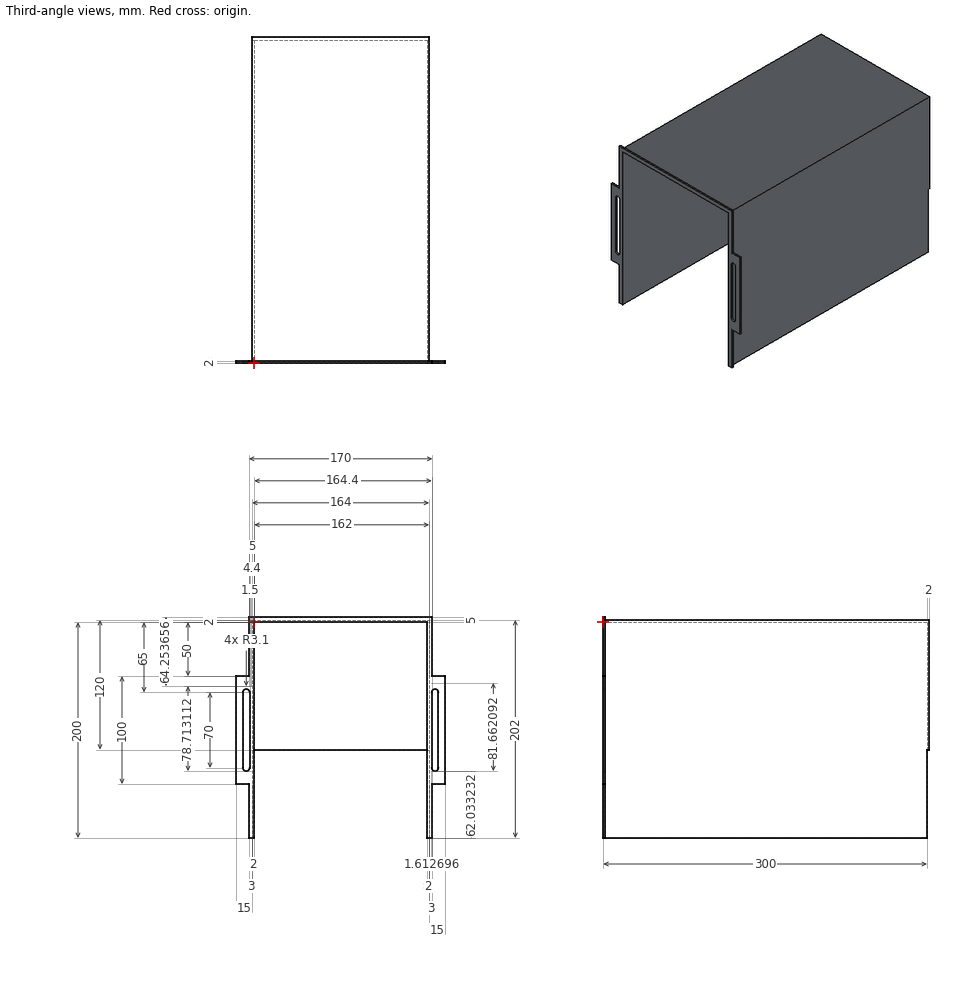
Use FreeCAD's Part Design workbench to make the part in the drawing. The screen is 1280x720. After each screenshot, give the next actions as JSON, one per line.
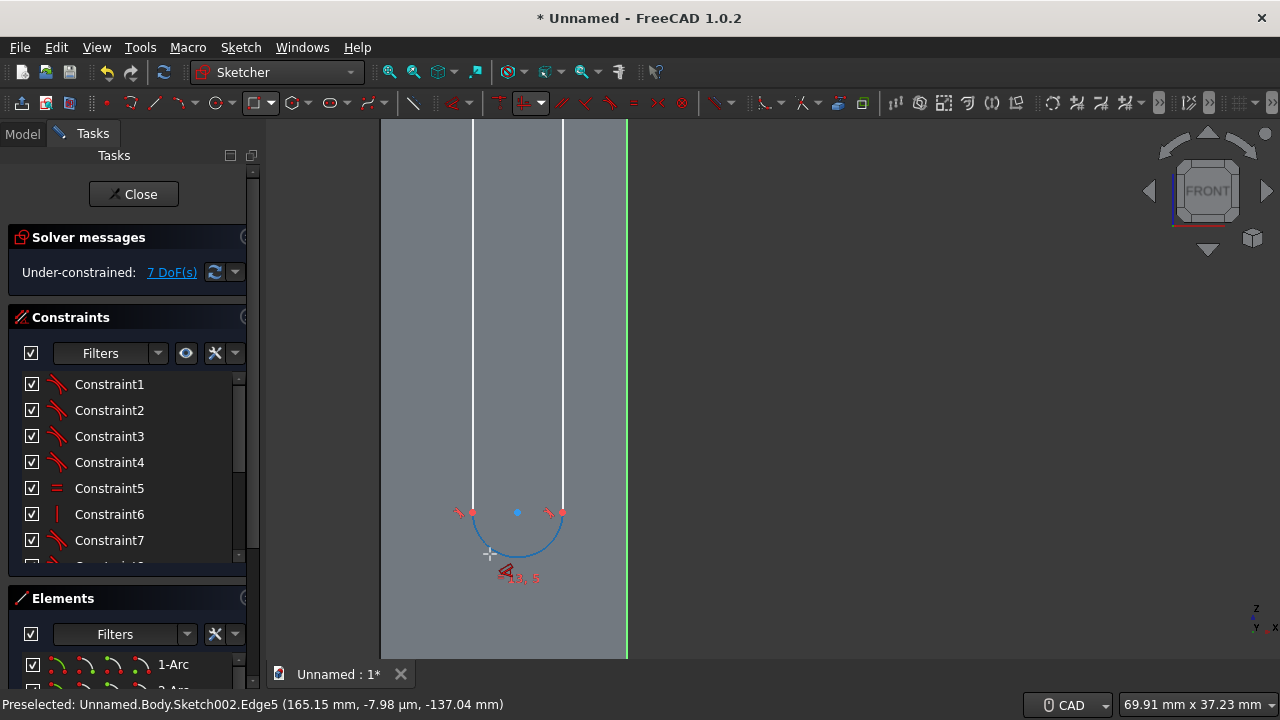
{"action": "left_click", "coordinate": [491, 549]}
{"action": "left_click", "coordinate": [472, 575]}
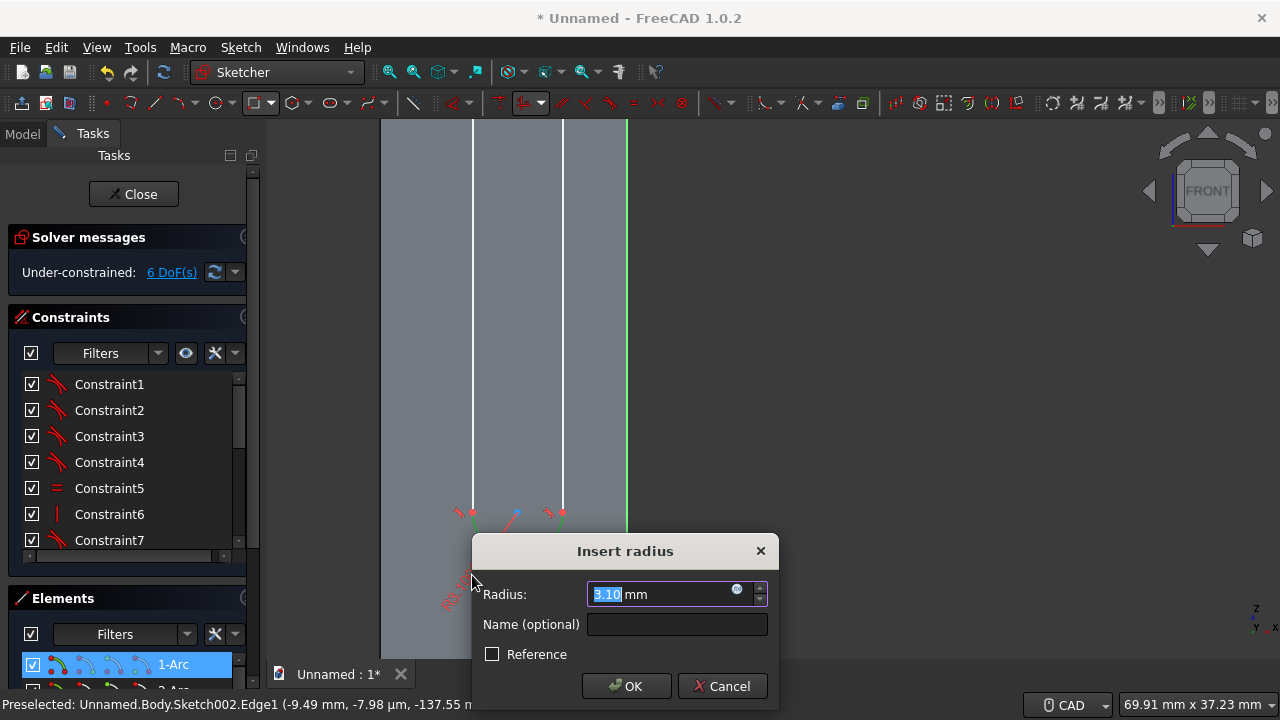
{"action": "type", "text": "3.1"}
{"action": "key", "text": "Return"}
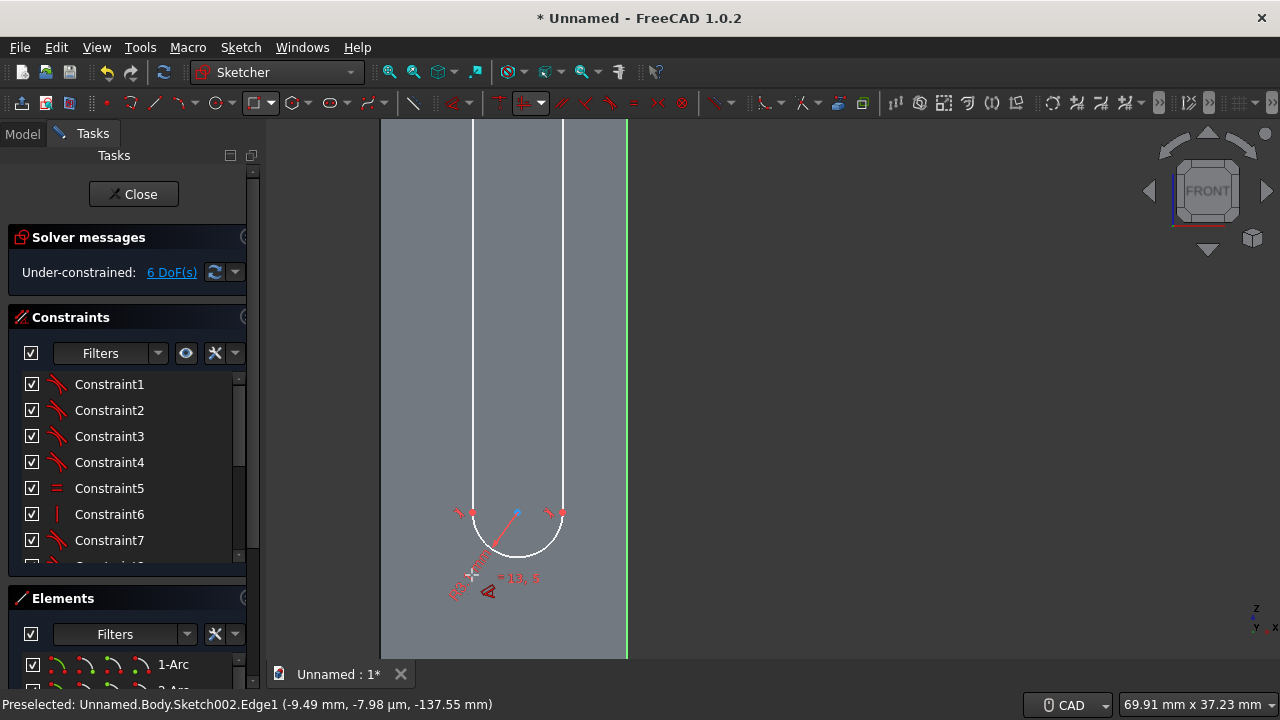
{"action": "scroll", "coordinate": [490, 554], "scroll_direction": "down", "scroll_amount": 9}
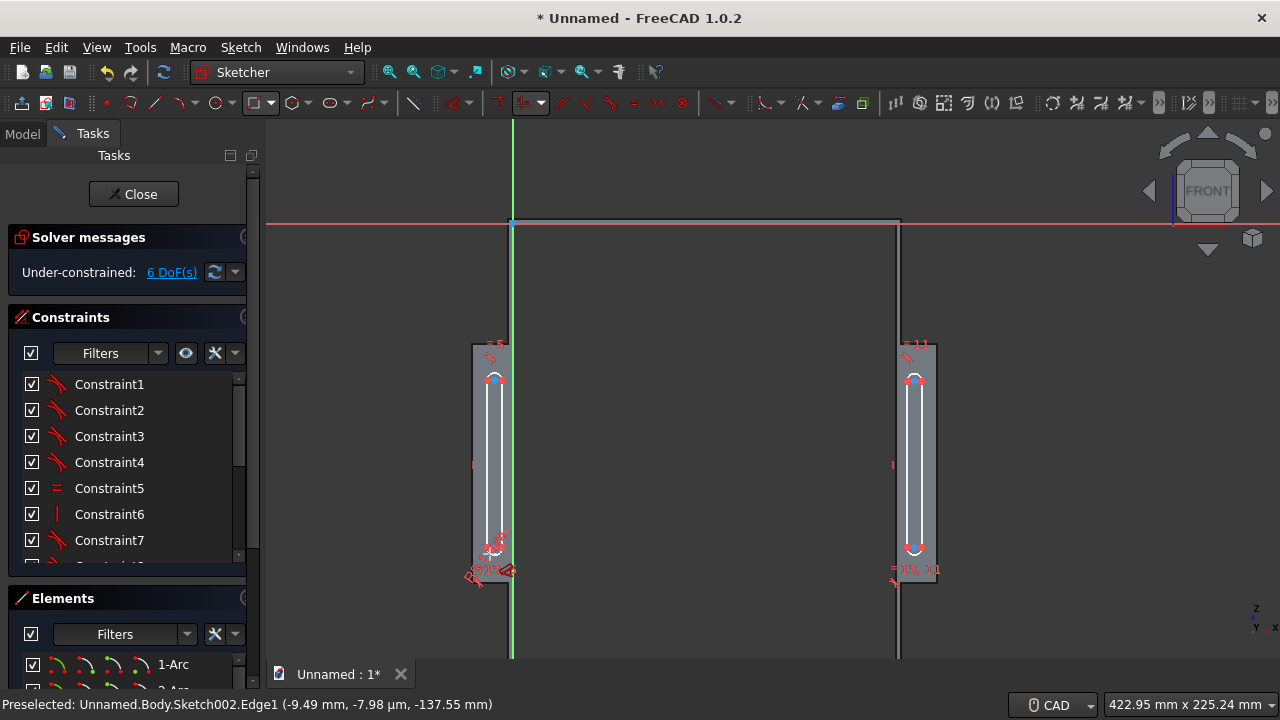
{"action": "left_click", "coordinate": [487, 498]}
{"action": "left_click", "coordinate": [453, 464]}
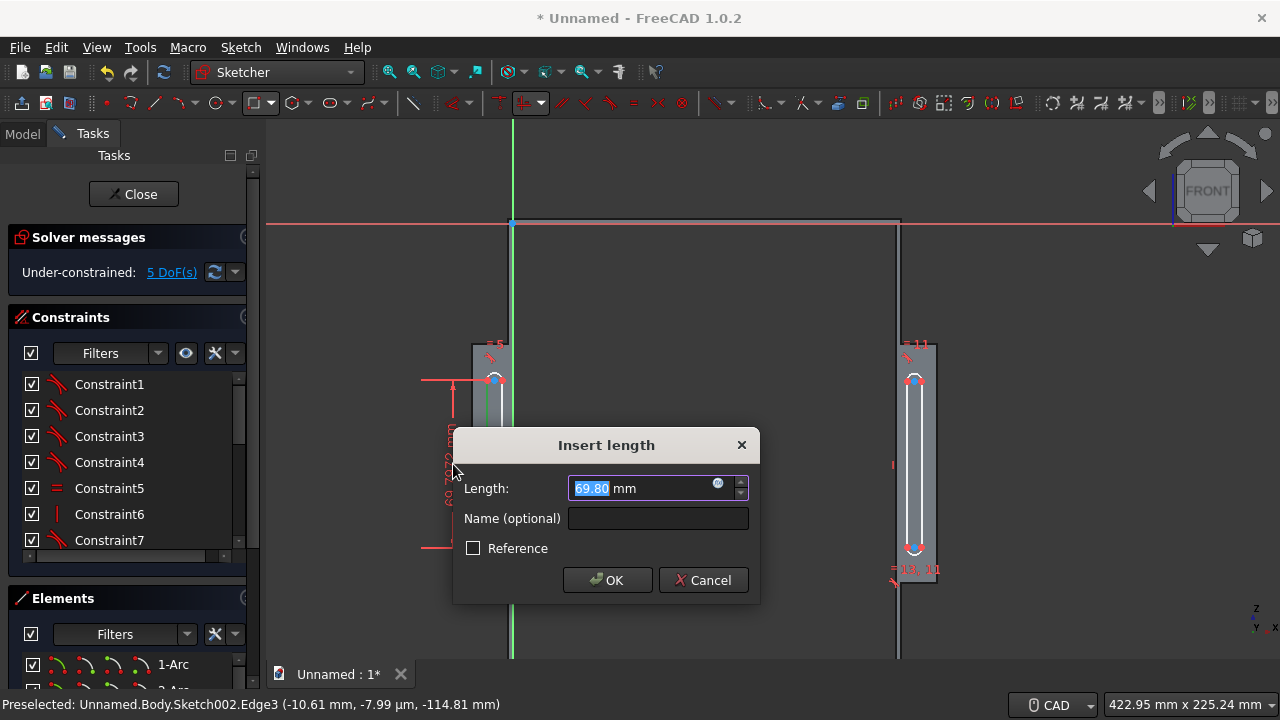
{"action": "type", "text": "70"}
{"action": "key", "text": "Return"}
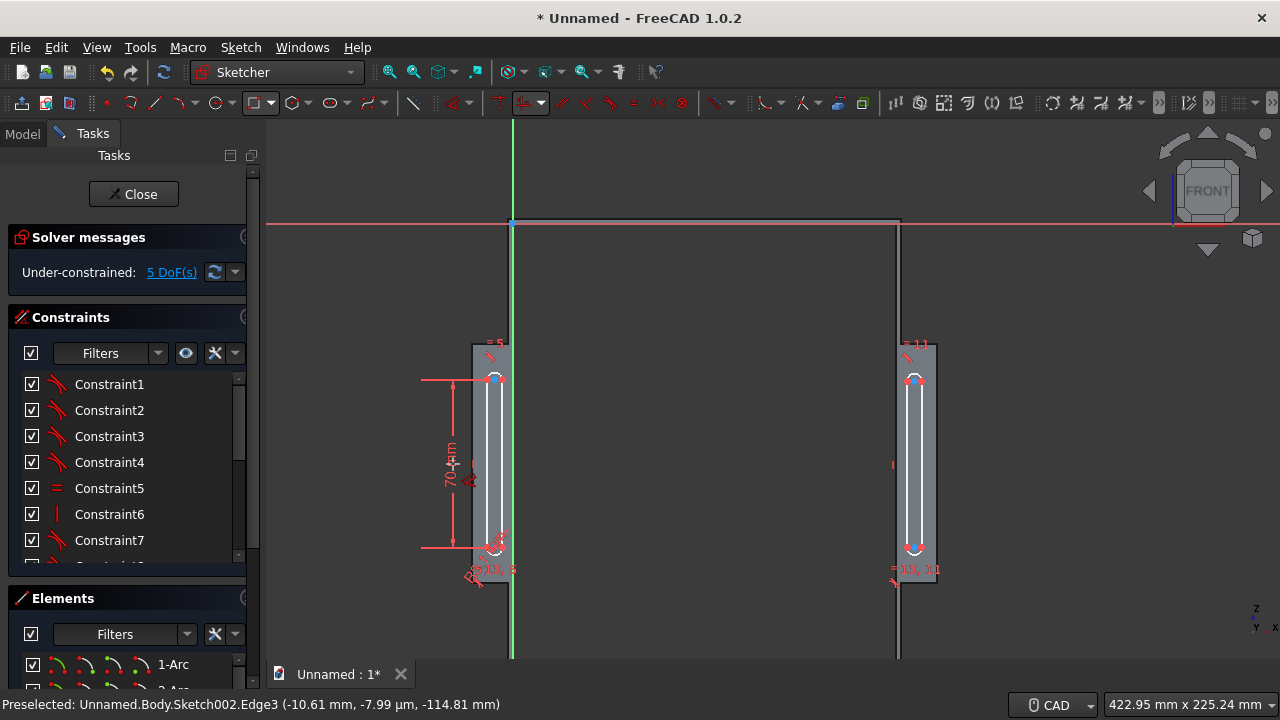
{"action": "left_click", "coordinate": [907, 498]}
{"action": "left_click", "coordinate": [941, 464]}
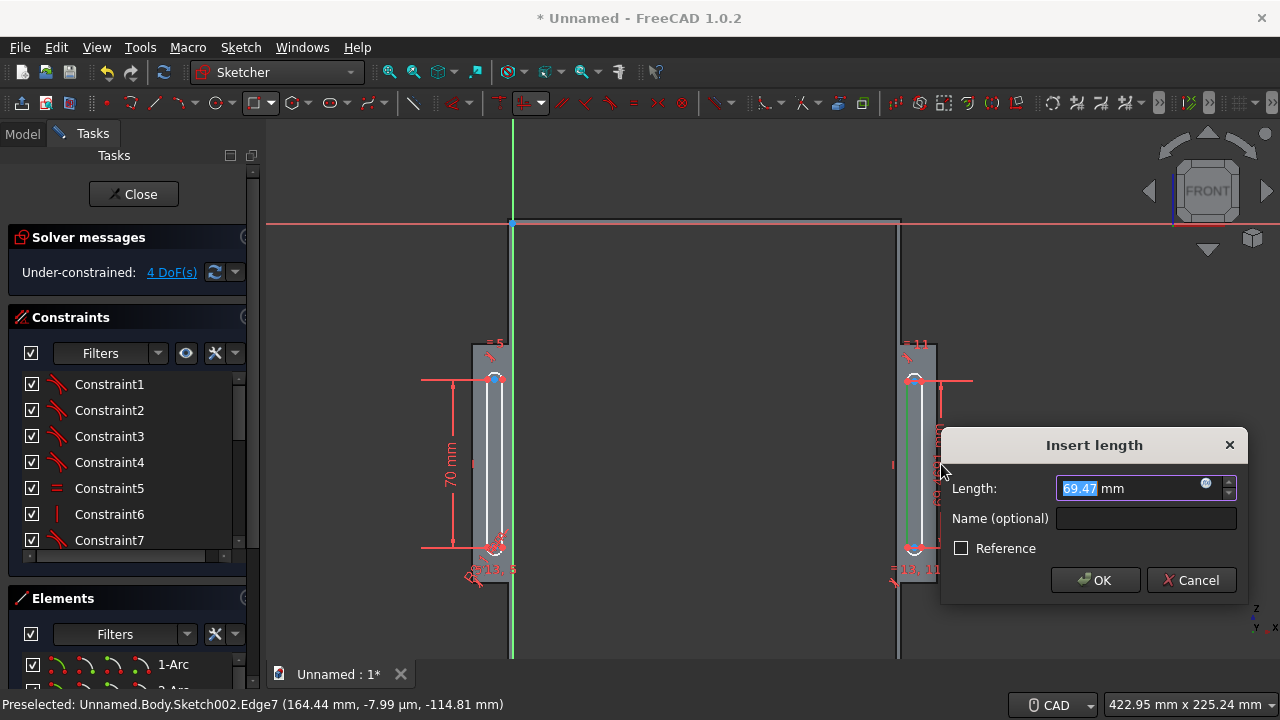
{"action": "type", "text": "70"}
{"action": "key", "text": "Return"}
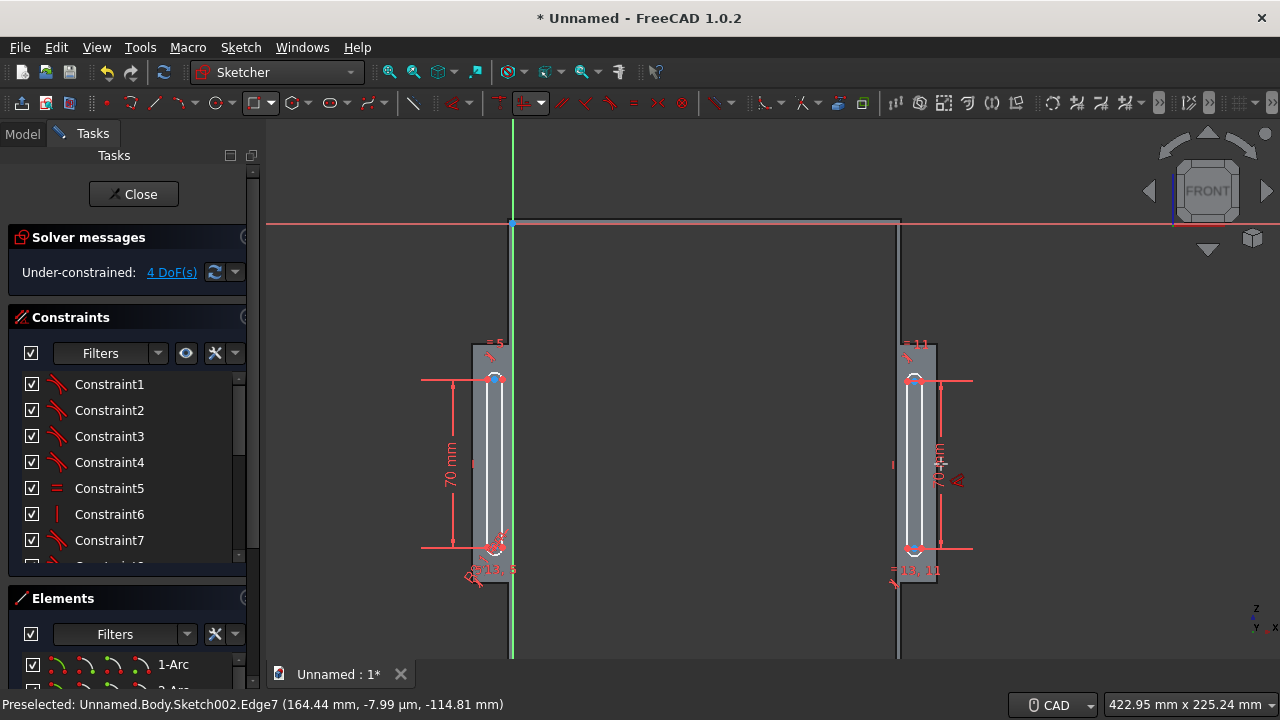
{"action": "scroll", "coordinate": [502, 380], "scroll_direction": "up", "scroll_amount": 3}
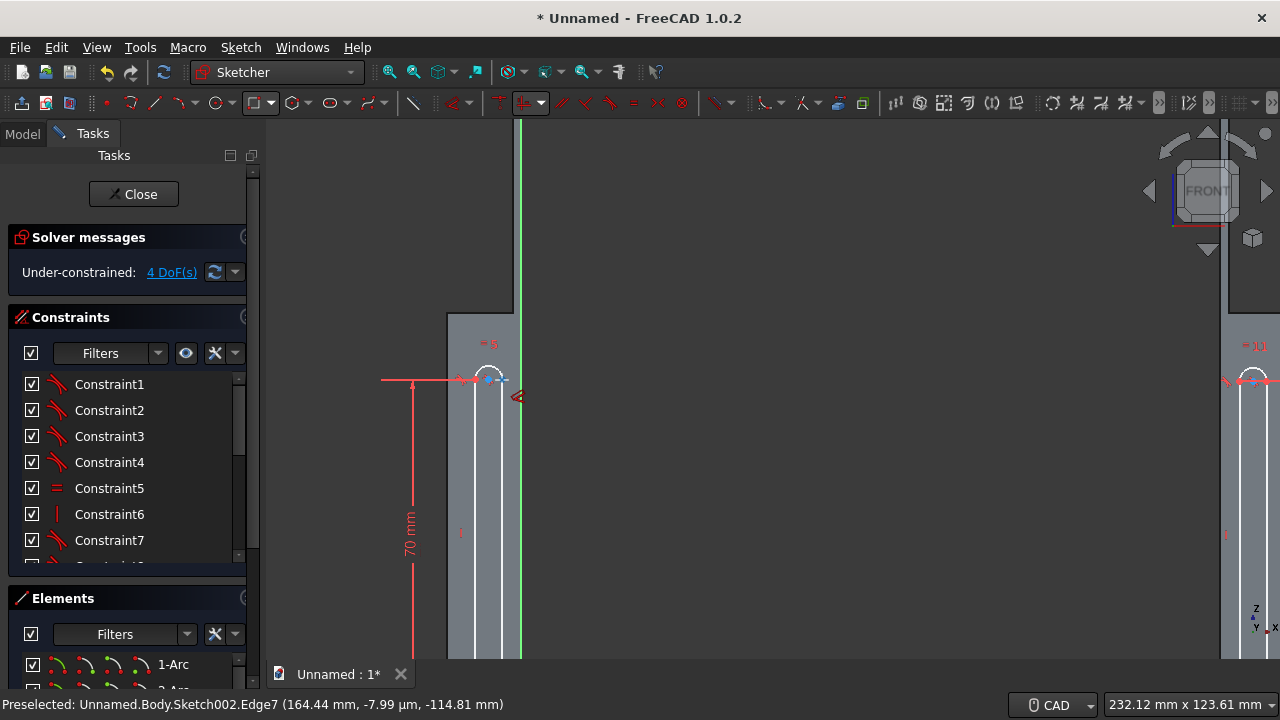
{"action": "left_click", "coordinate": [502, 380]}
{"action": "left_click", "coordinate": [468, 263]}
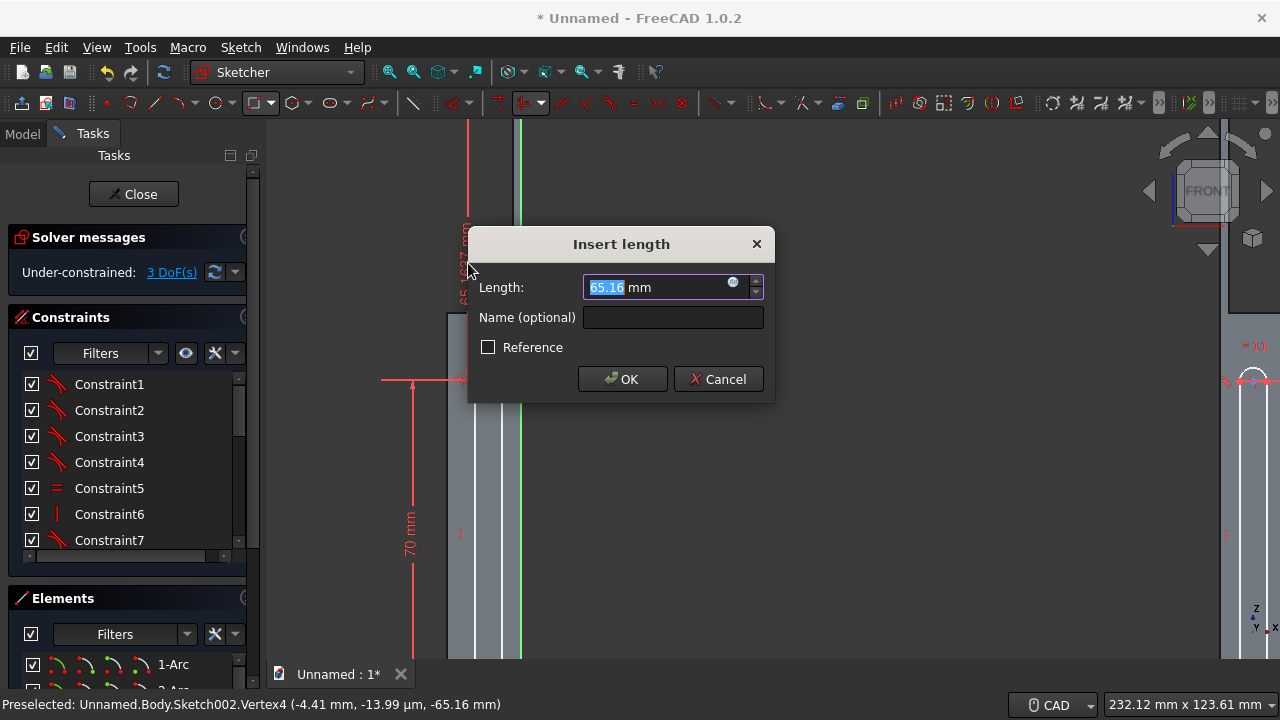
{"action": "type", "text": "65"}
{"action": "key", "text": "Return"}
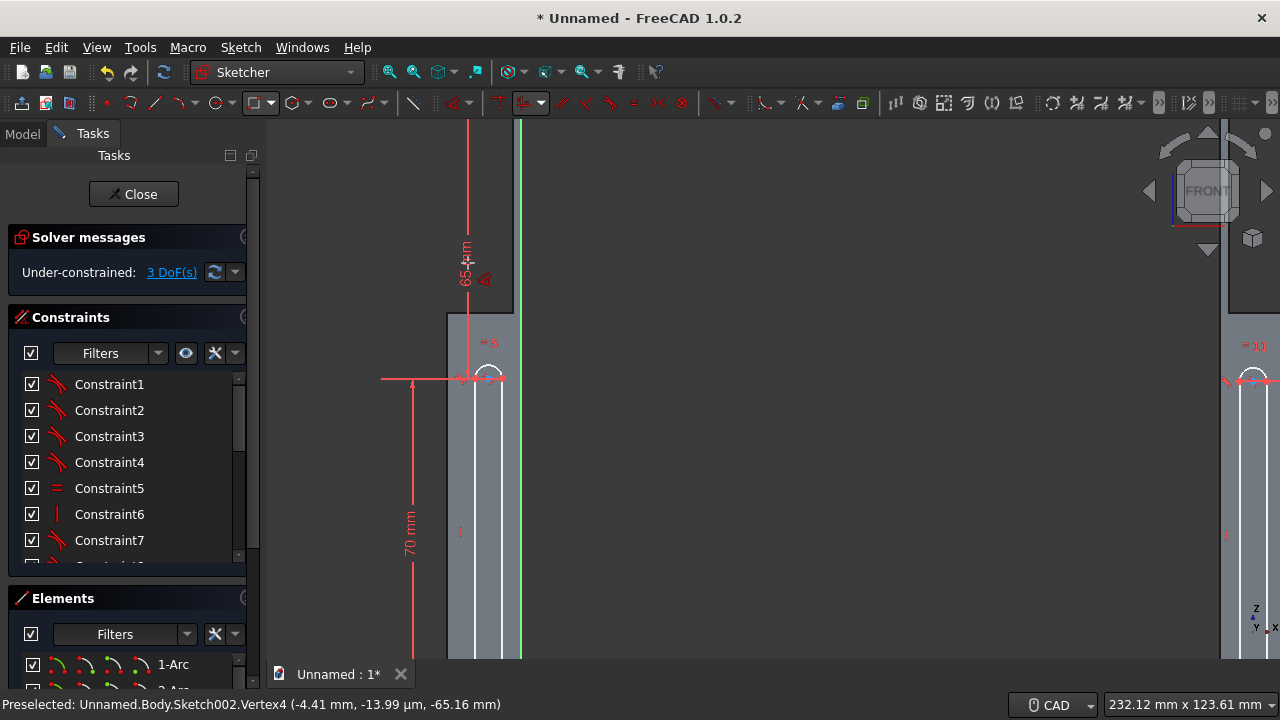
{"action": "scroll", "coordinate": [502, 380], "scroll_direction": "down", "scroll_amount": 3}